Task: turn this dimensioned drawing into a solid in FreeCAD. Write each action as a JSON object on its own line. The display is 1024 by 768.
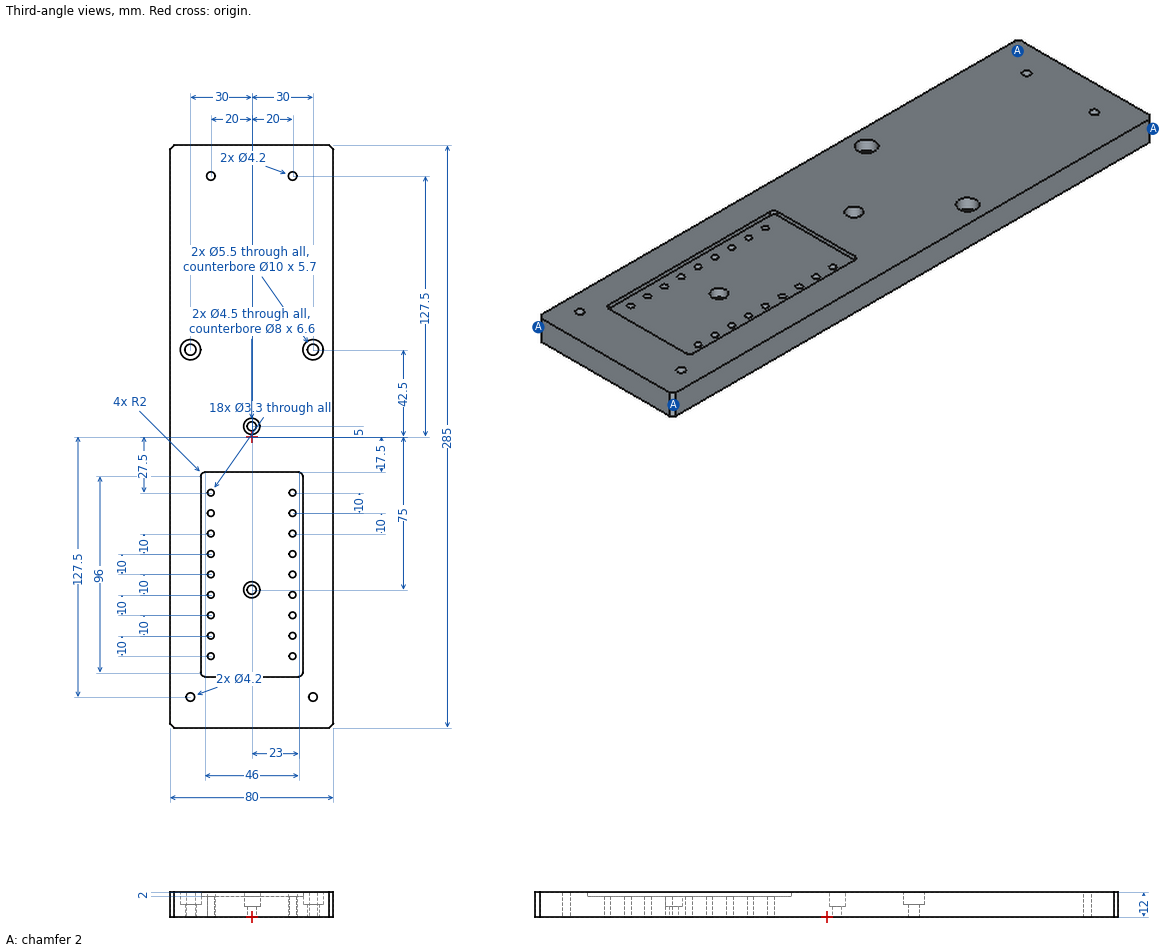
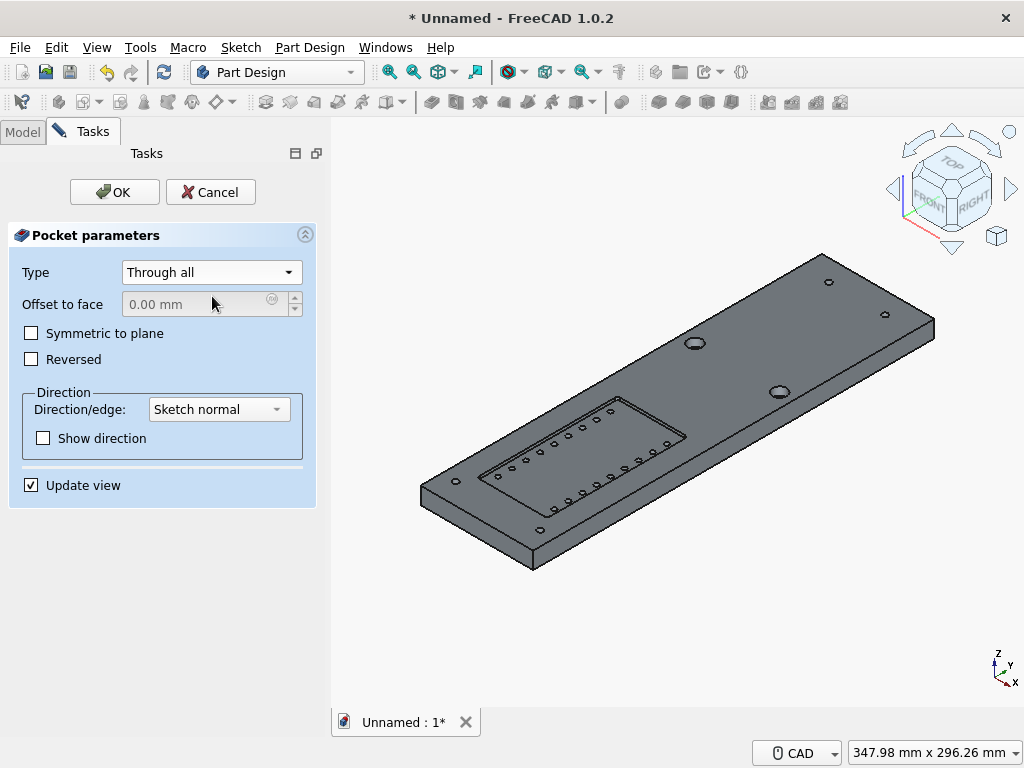
{"action": "left_click", "coordinate": [115, 192]}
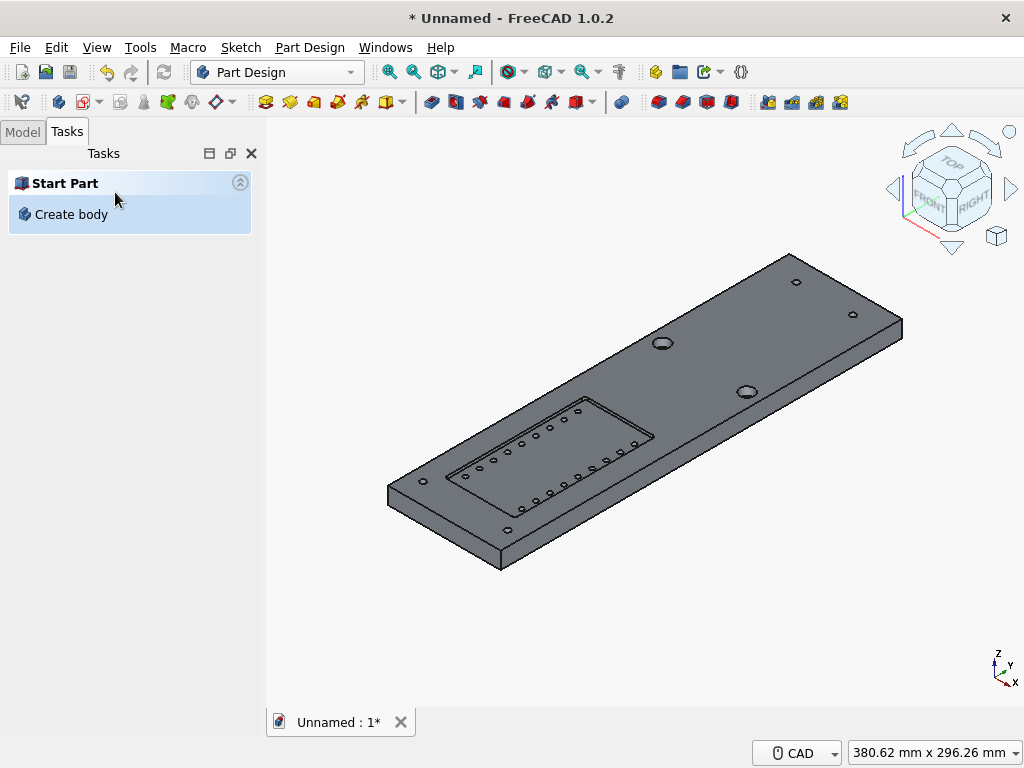
{"action": "left_click", "coordinate": [501, 559]}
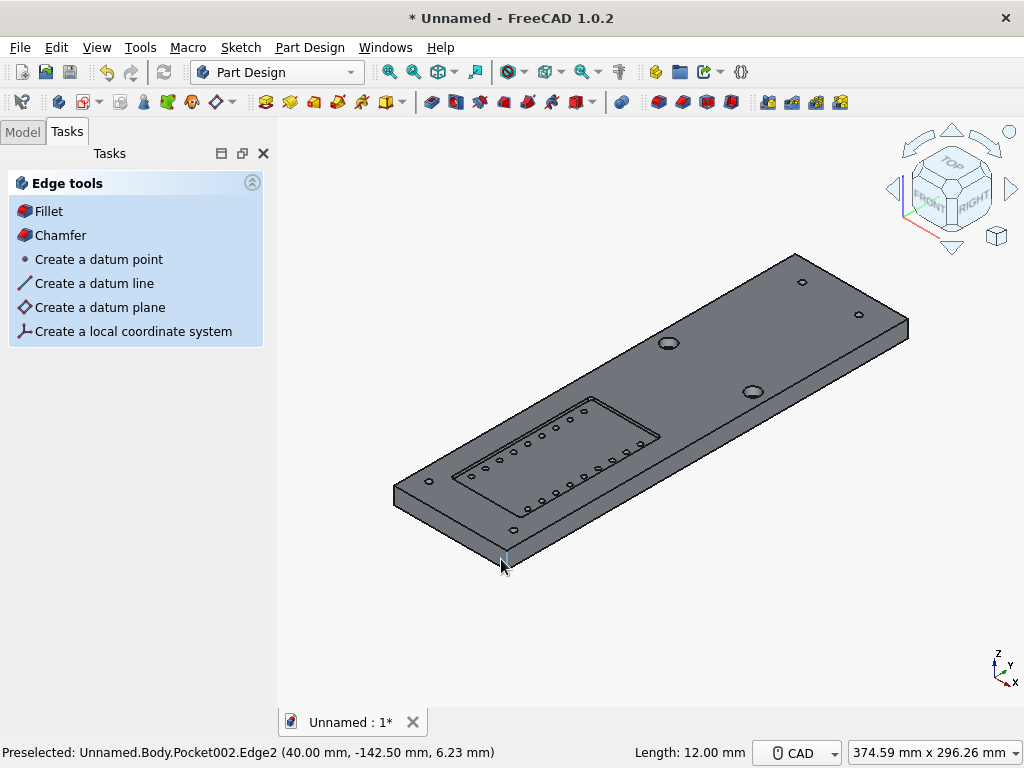
{"action": "key", "text": "2"}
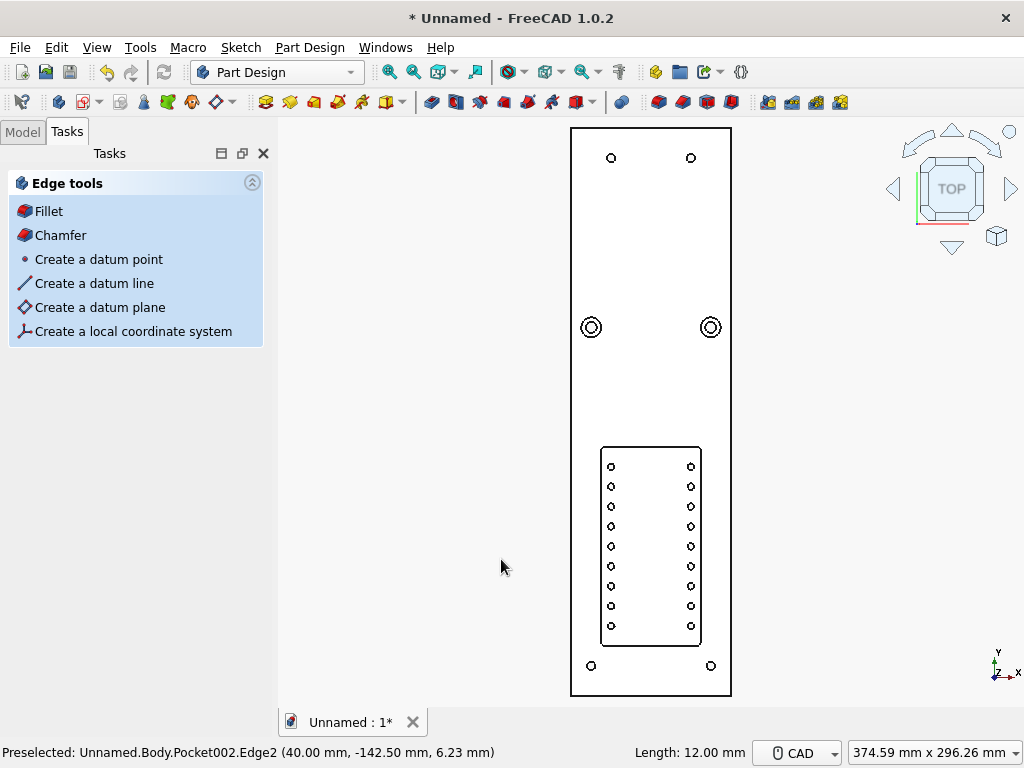
{"action": "key", "text": "0"}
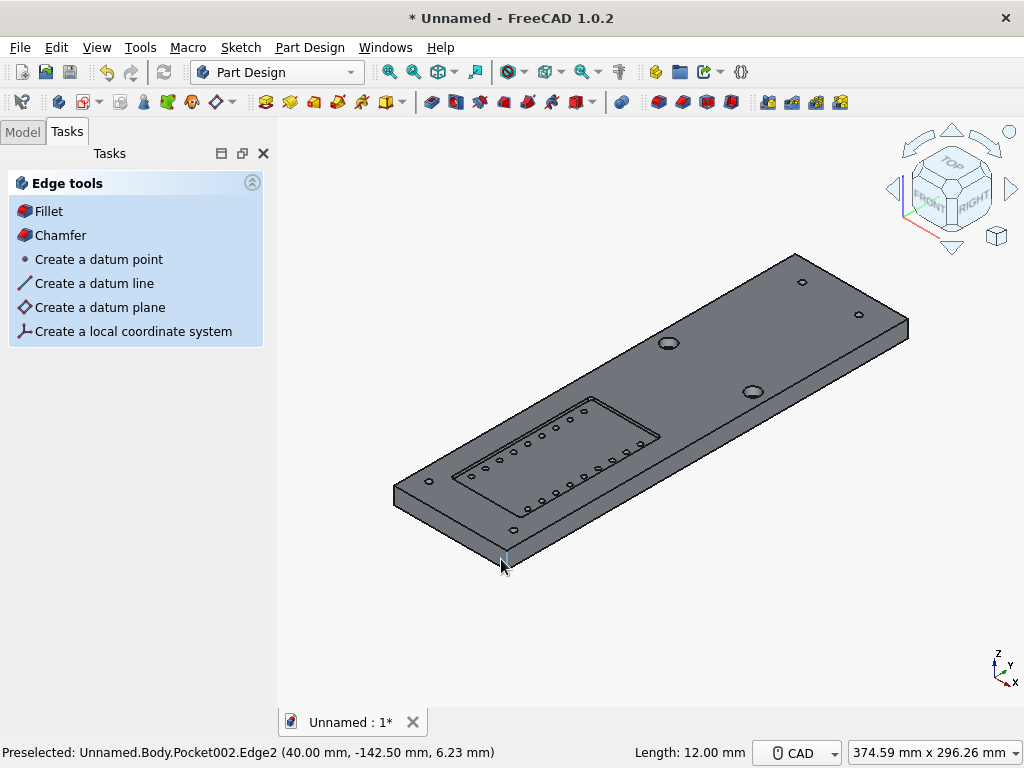
{"action": "key", "text": "1"}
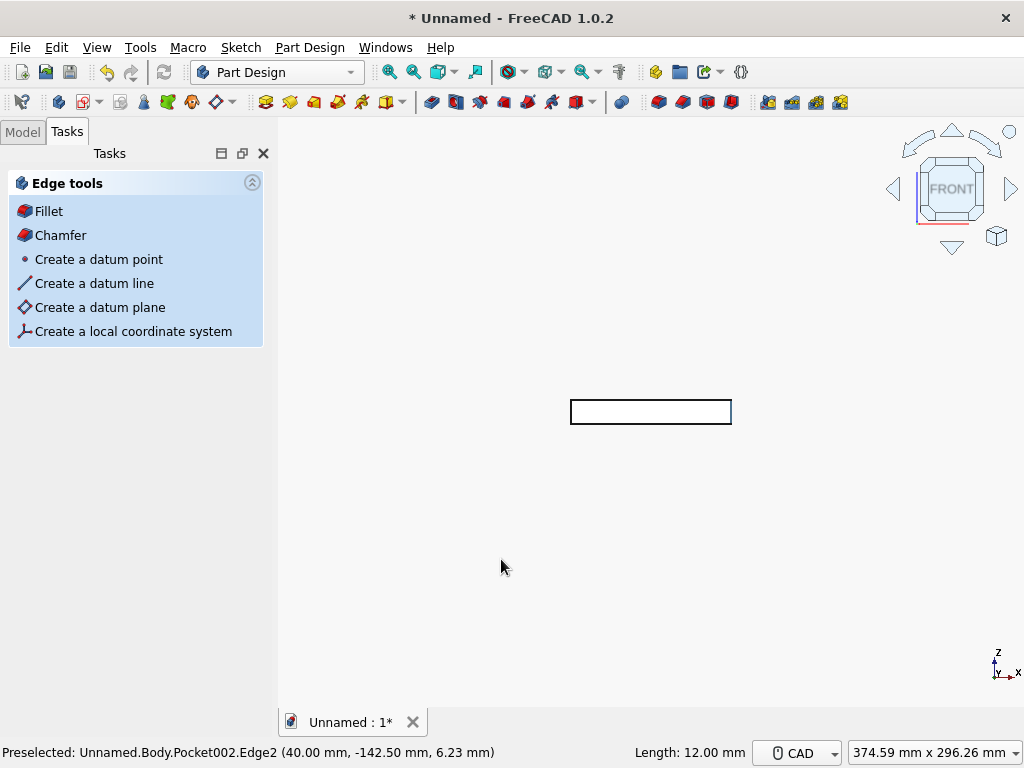
{"action": "key", "text": "v f"}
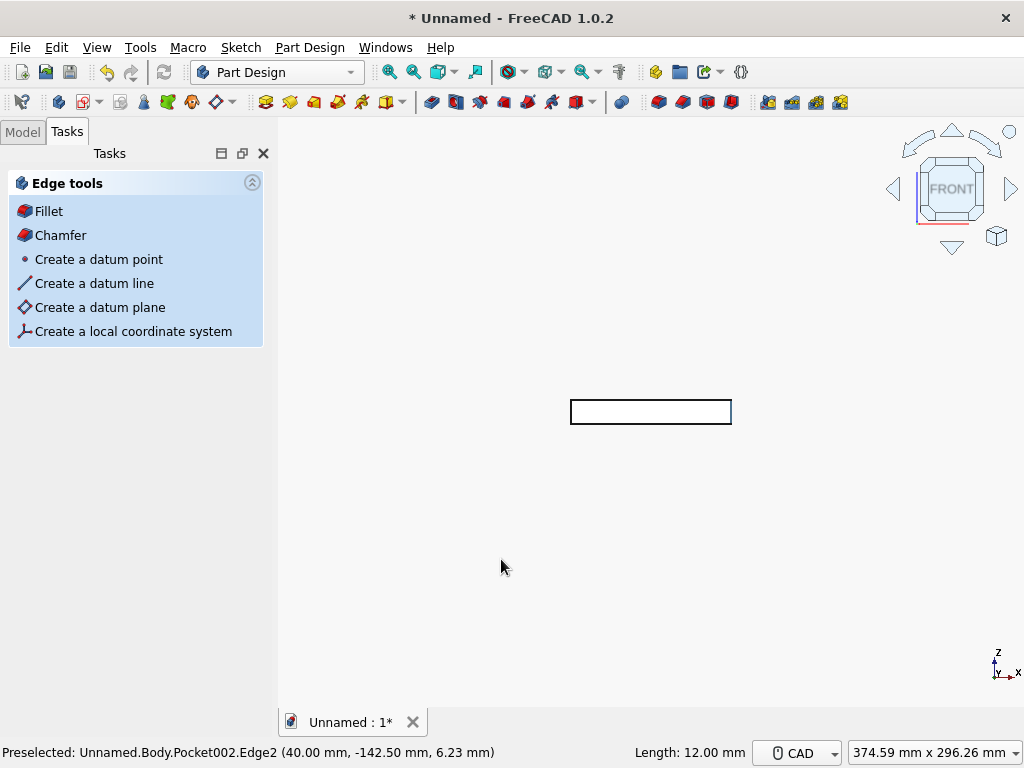
{"action": "left_click", "coordinate": [571, 411], "text": "ctrl"}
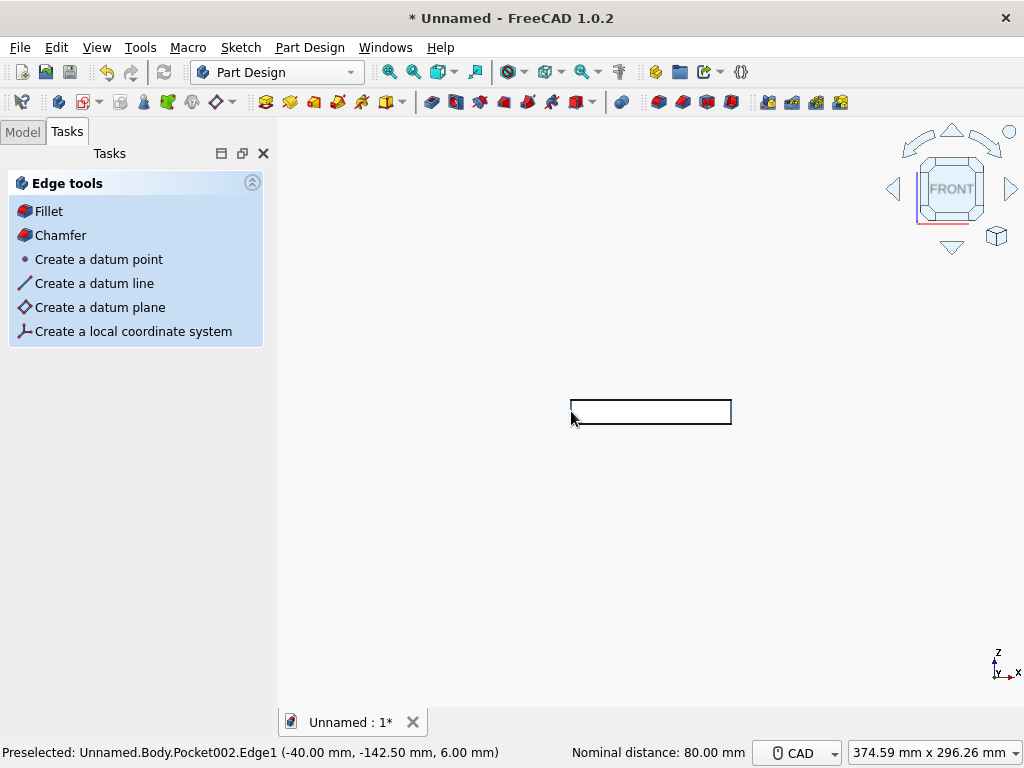
{"action": "key", "text": "3"}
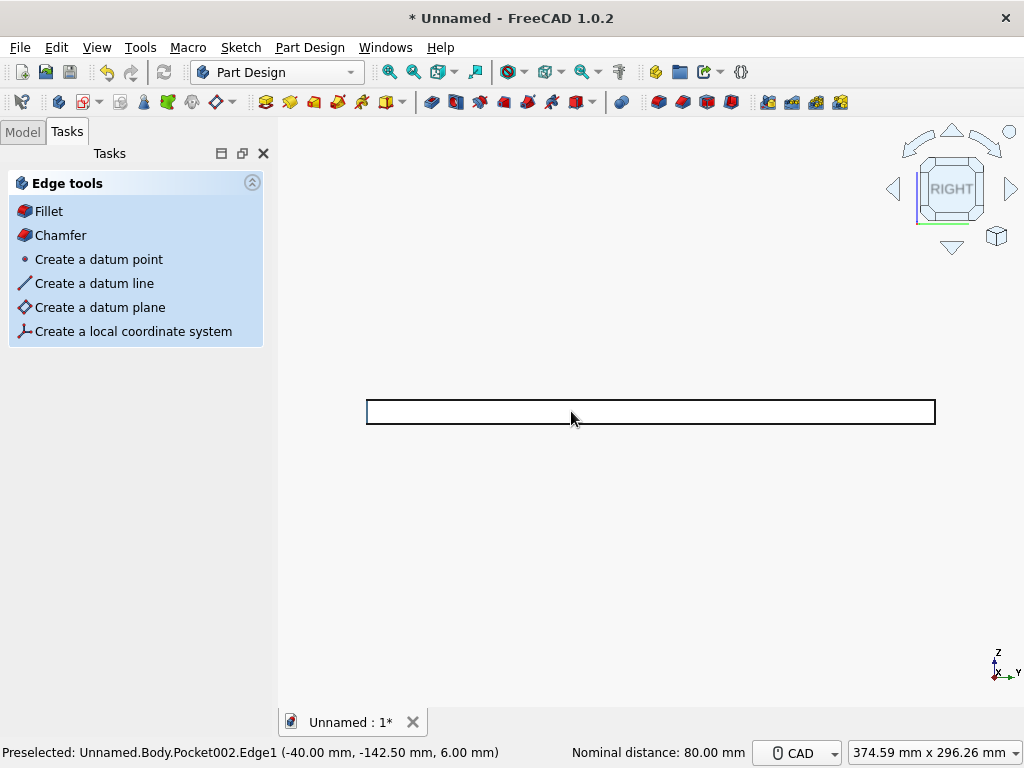
{"action": "left_click", "coordinate": [935, 411], "text": "ctrl"}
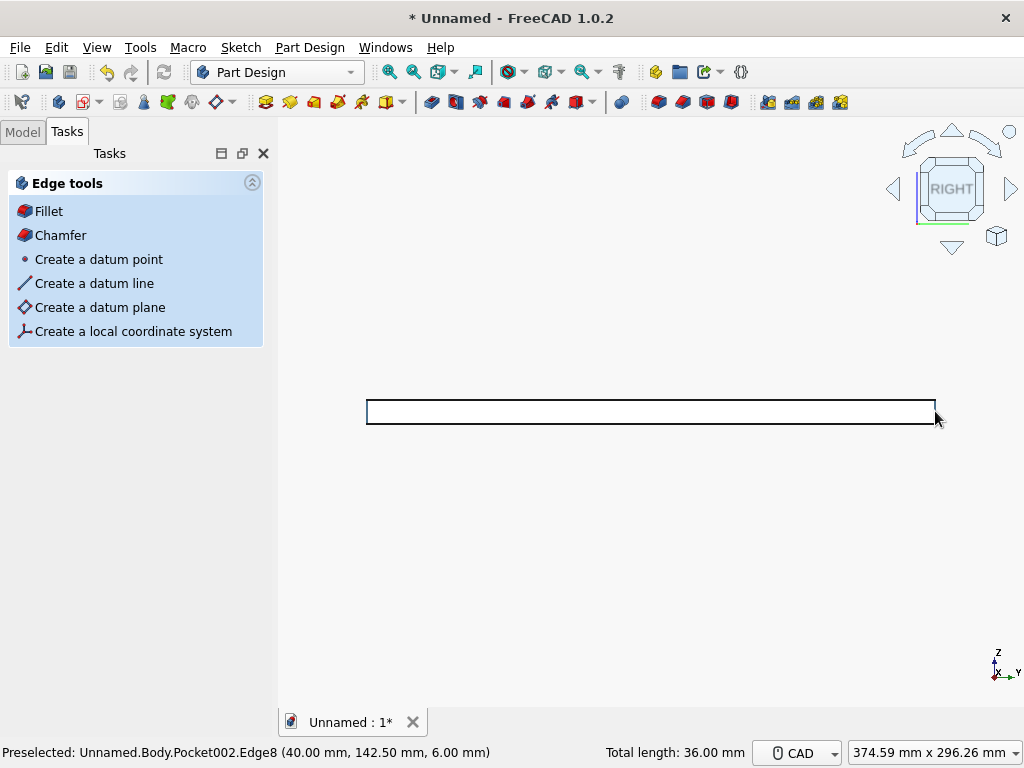
{"action": "key", "text": "5"}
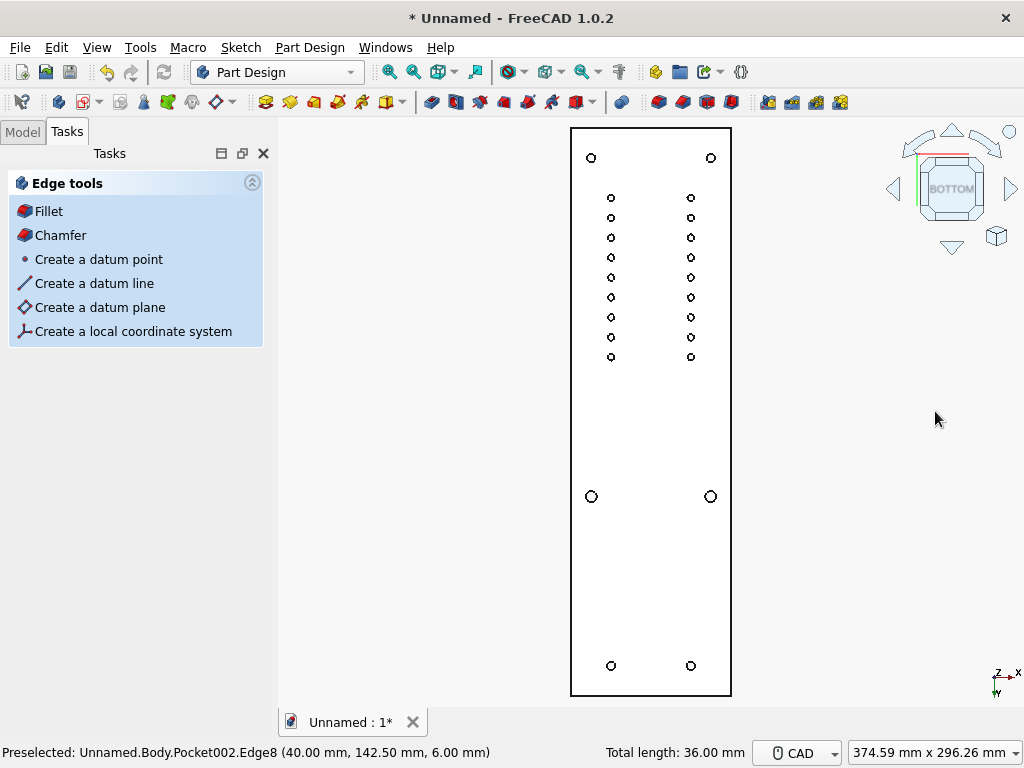
{"action": "key", "text": "4"}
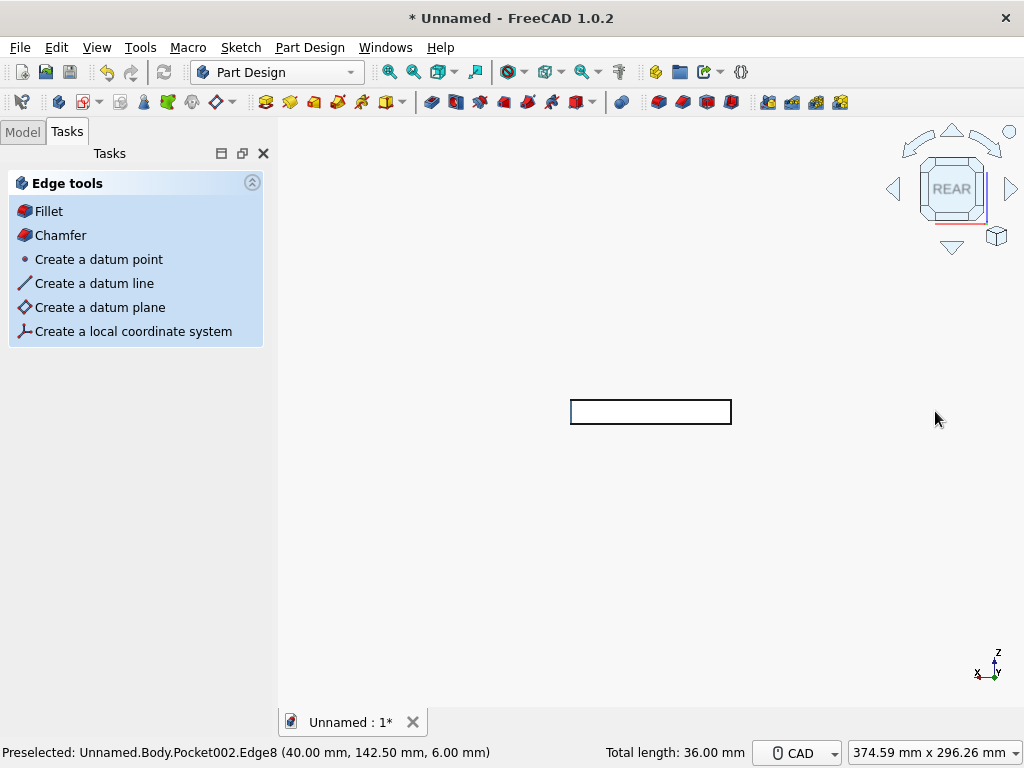
{"action": "key", "text": "v f"}